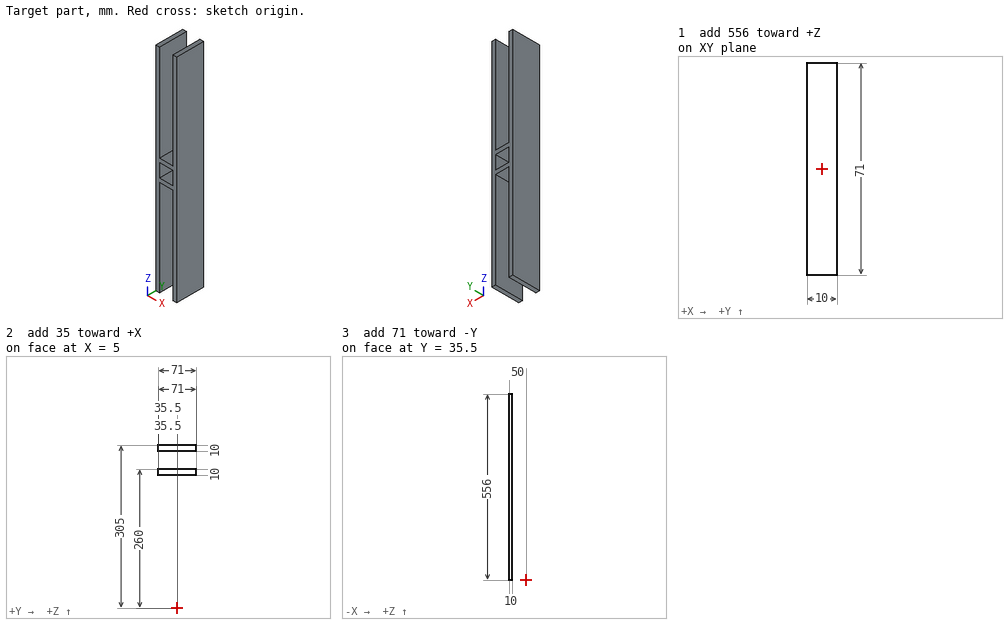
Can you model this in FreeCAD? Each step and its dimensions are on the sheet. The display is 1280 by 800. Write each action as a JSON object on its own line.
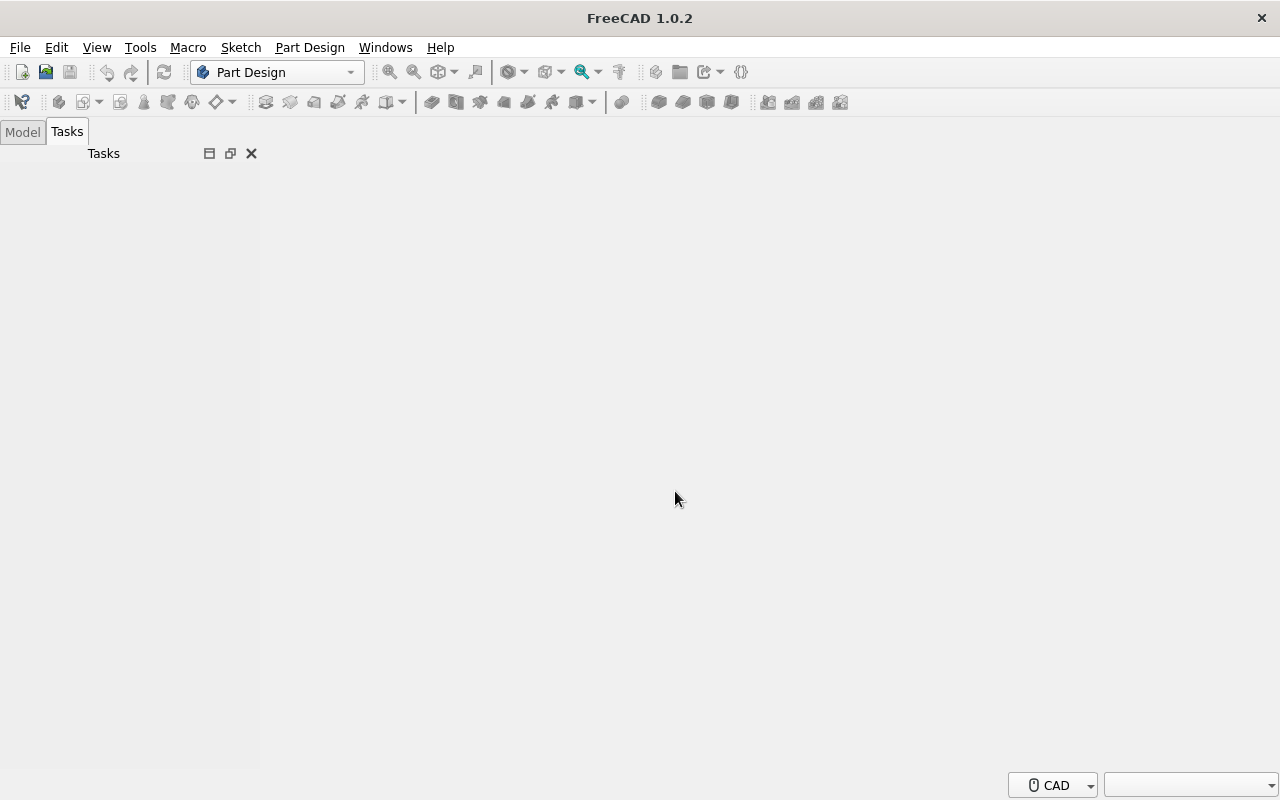
{"action": "left_click", "coordinate": [22, 72]}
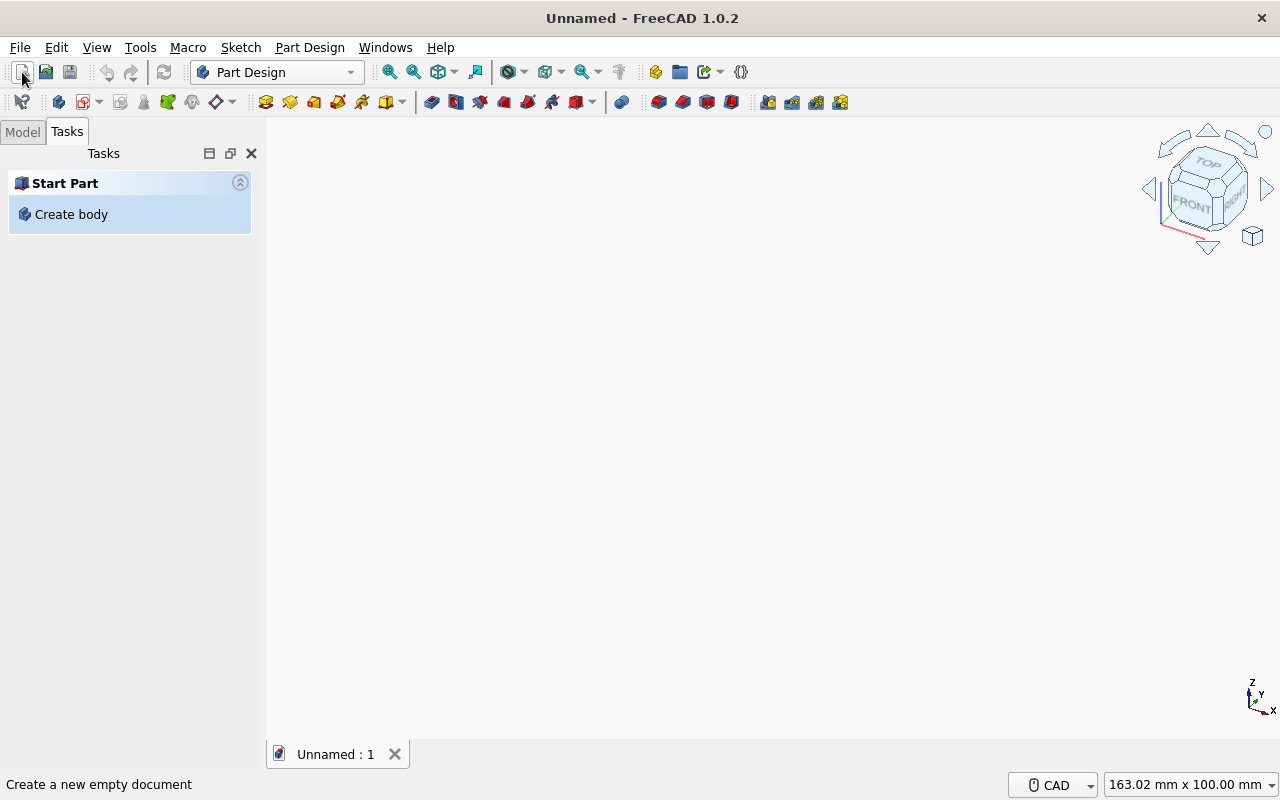
{"action": "left_click", "coordinate": [84, 102]}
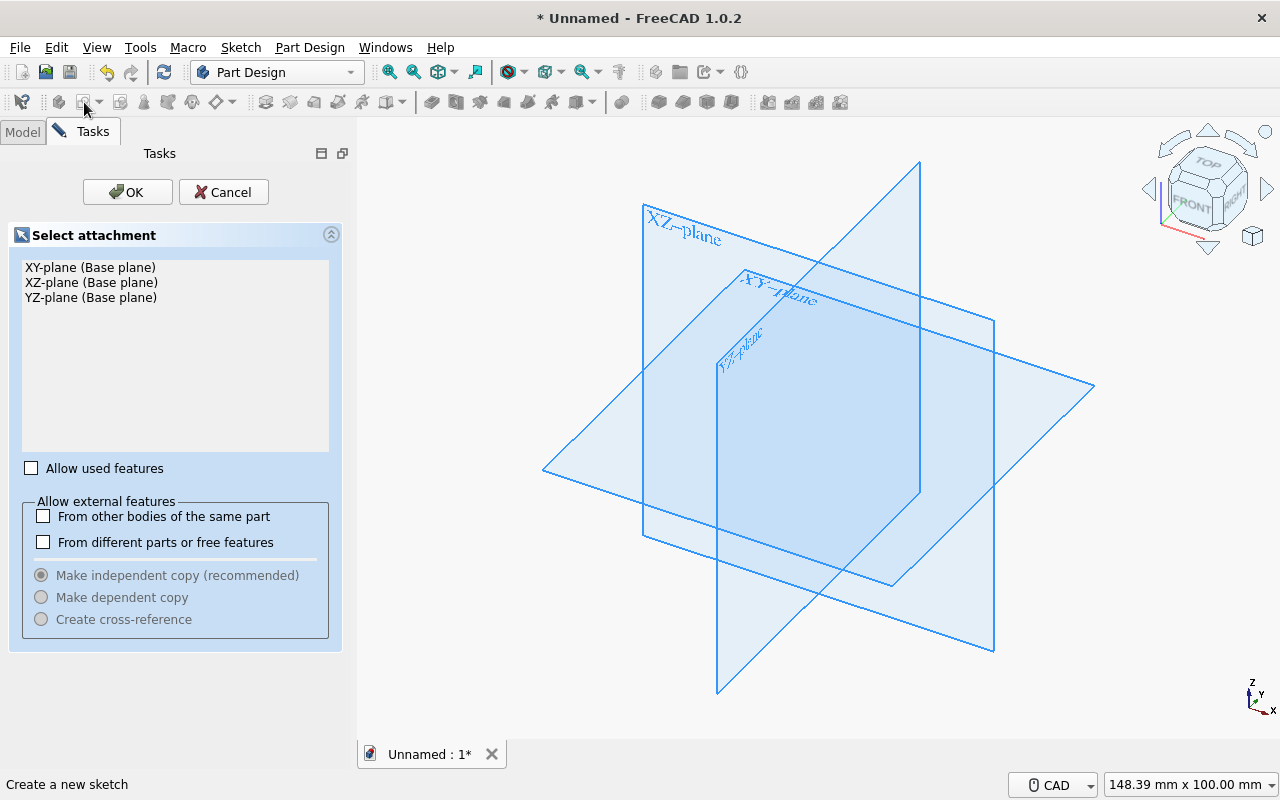
{"action": "left_click", "coordinate": [82, 268]}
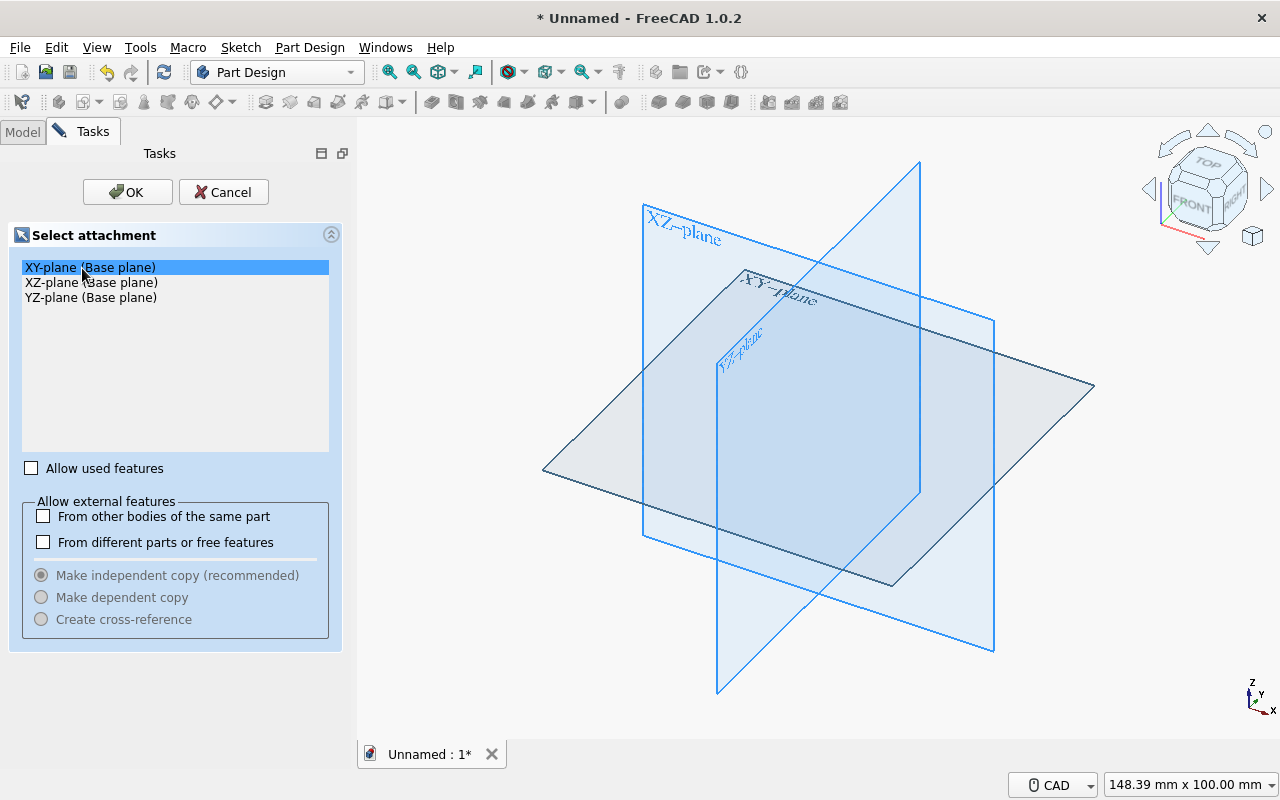
{"action": "left_click", "coordinate": [128, 192]}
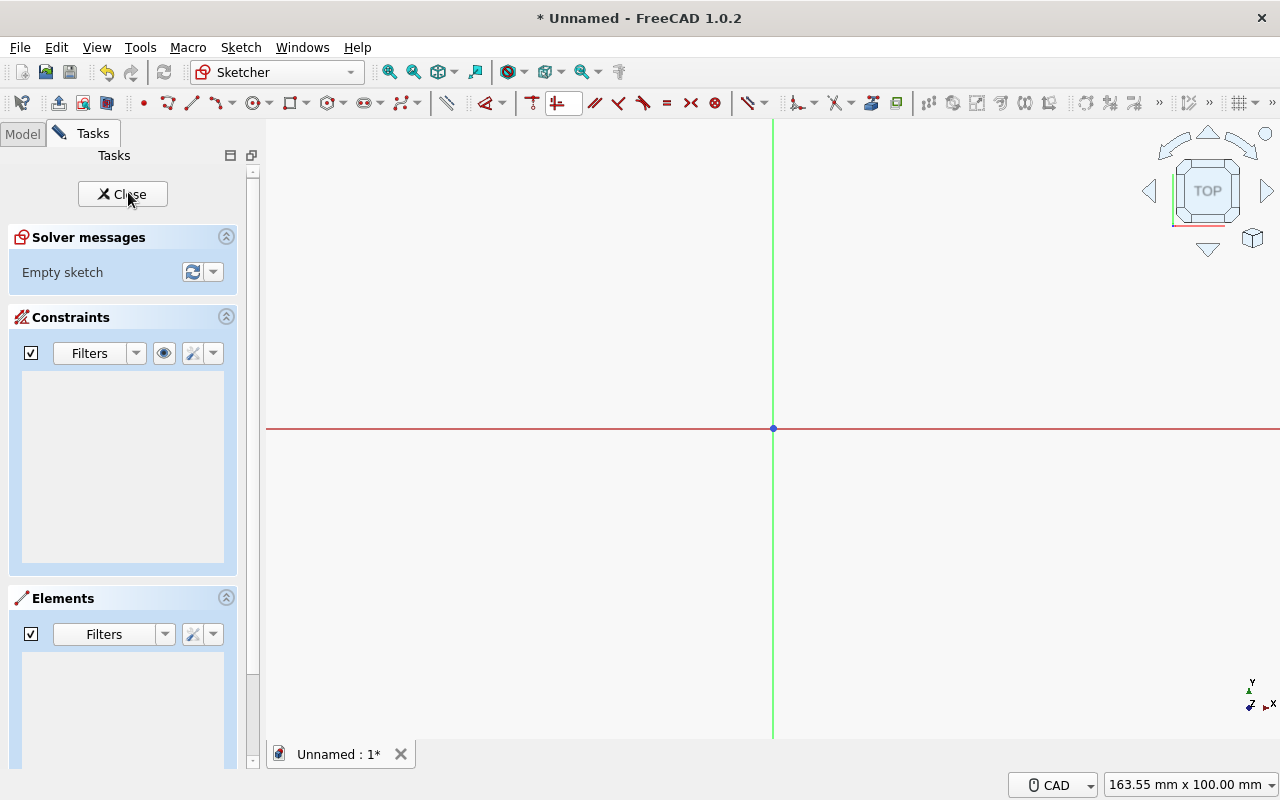
{"action": "left_click", "coordinate": [308, 104]}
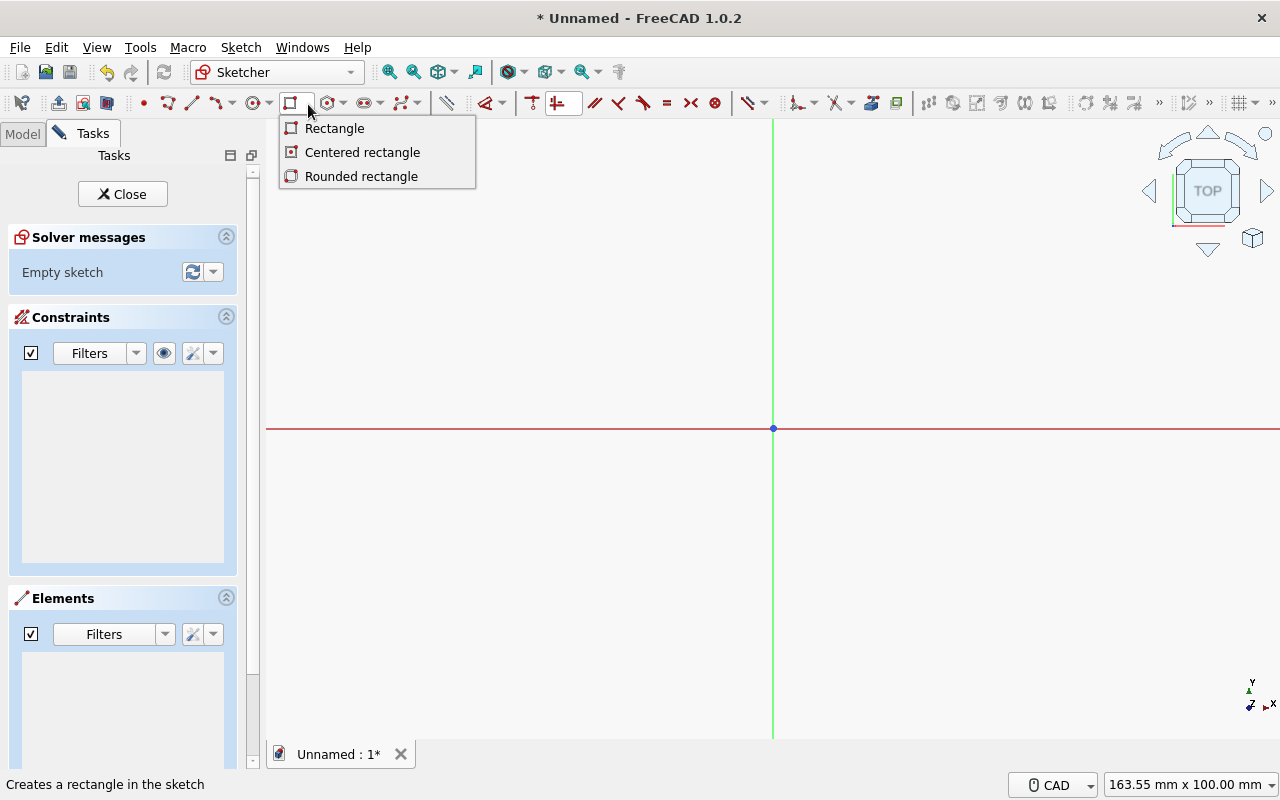
{"action": "left_click", "coordinate": [378, 152]}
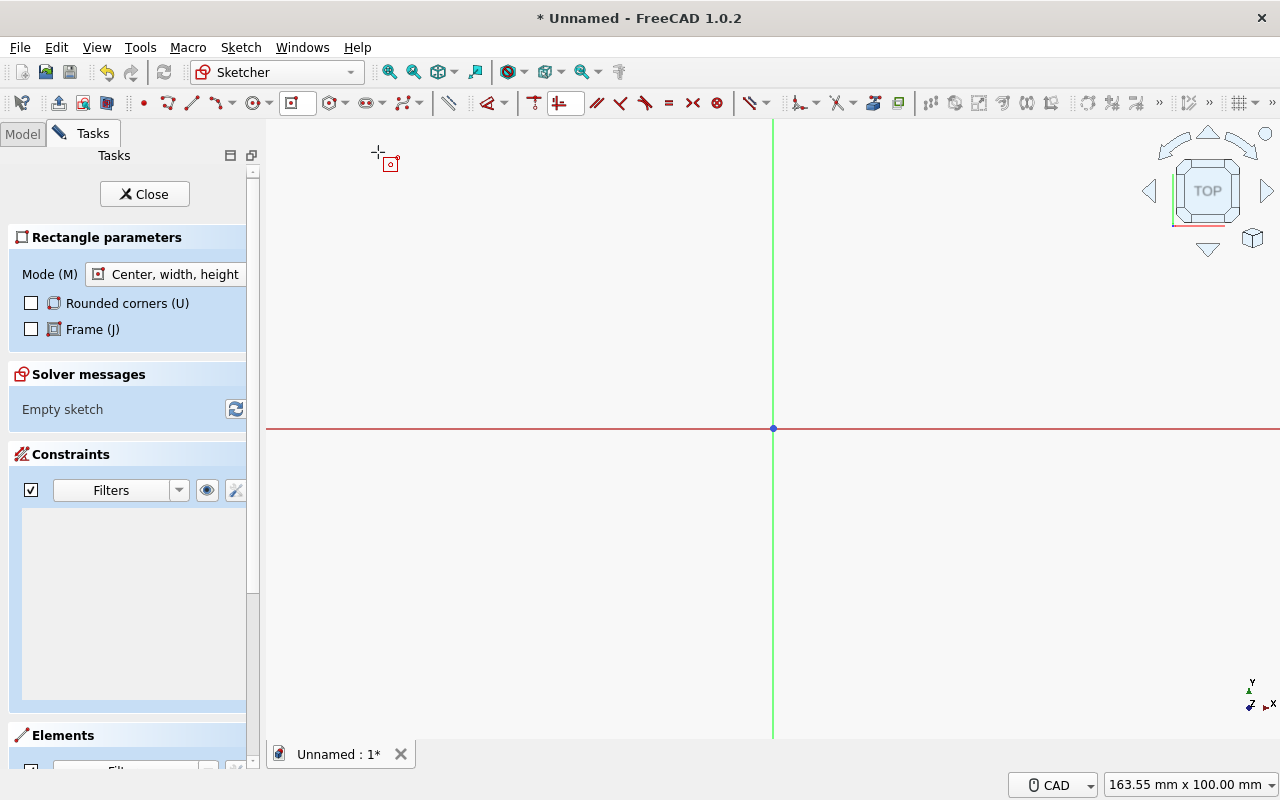
{"action": "left_click", "coordinate": [773, 429]}
{"action": "mouse_move", "coordinate": [804, 209]}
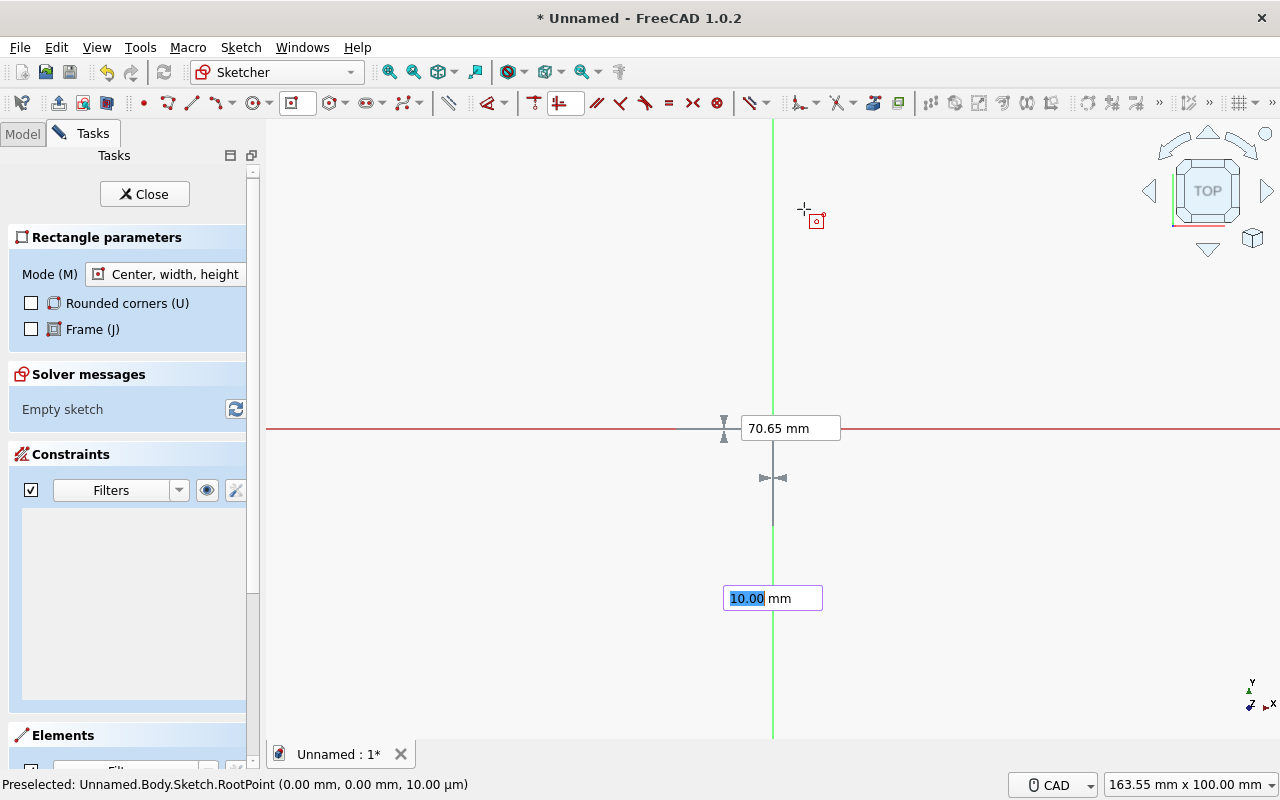
{"action": "type", "text": "10"}
{"action": "key", "text": "Tab"}
{"action": "type", "text": "71"}
{"action": "key", "text": "Return"}
{"action": "key", "text": "Escape"}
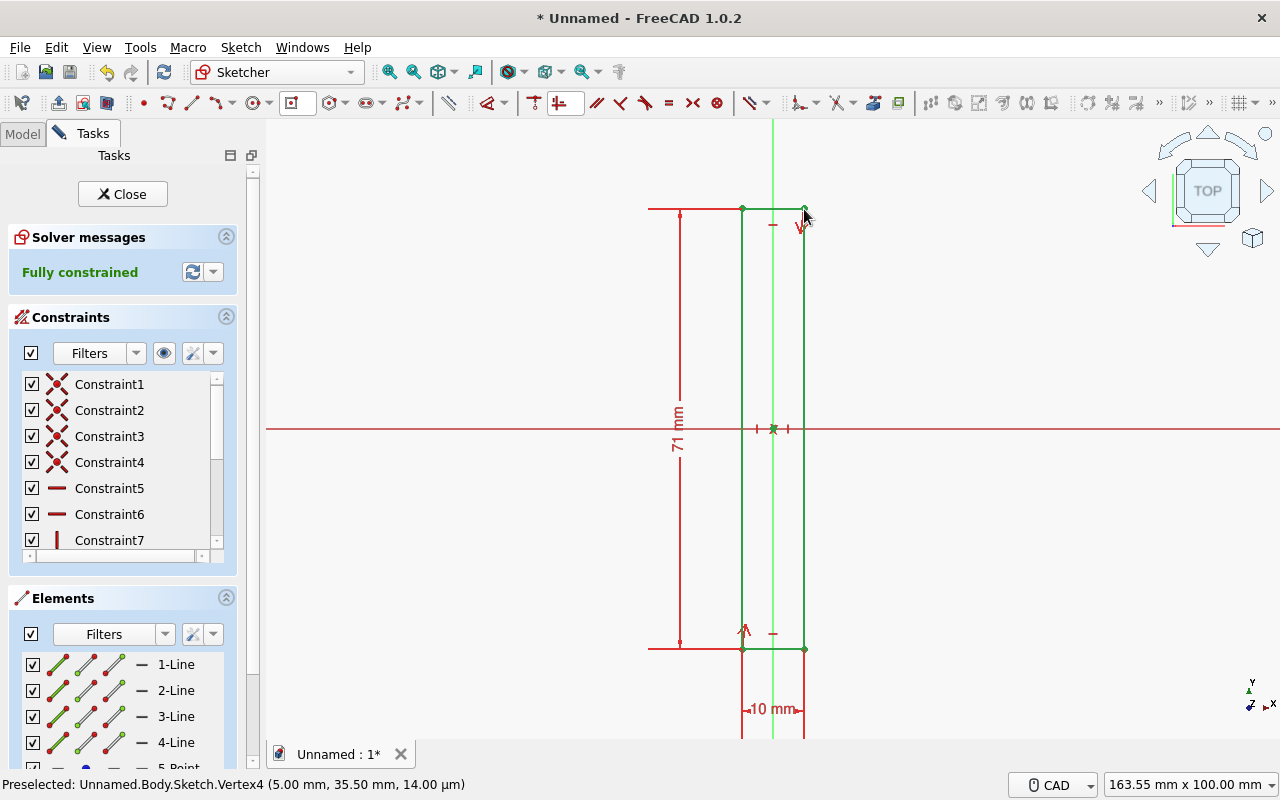
{"action": "left_click", "coordinate": [123, 194]}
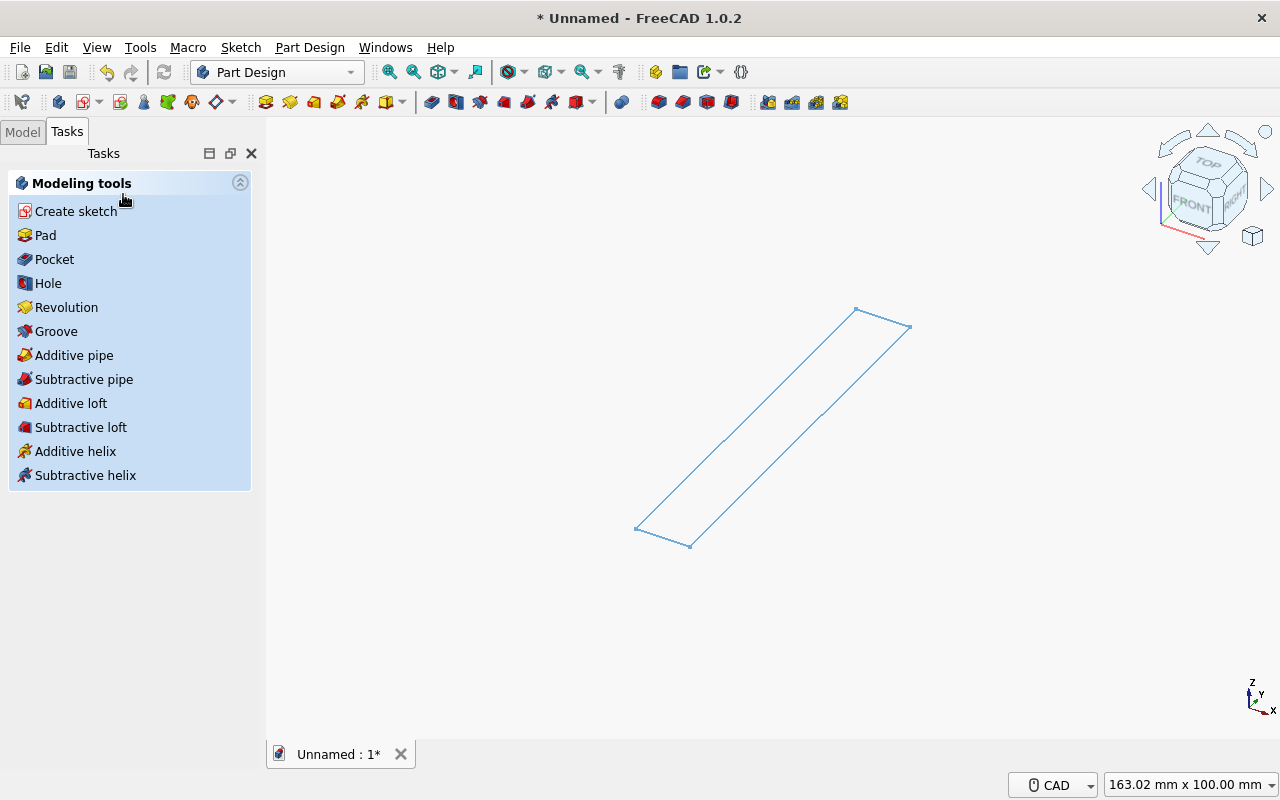
{"action": "left_click", "coordinate": [266, 102]}